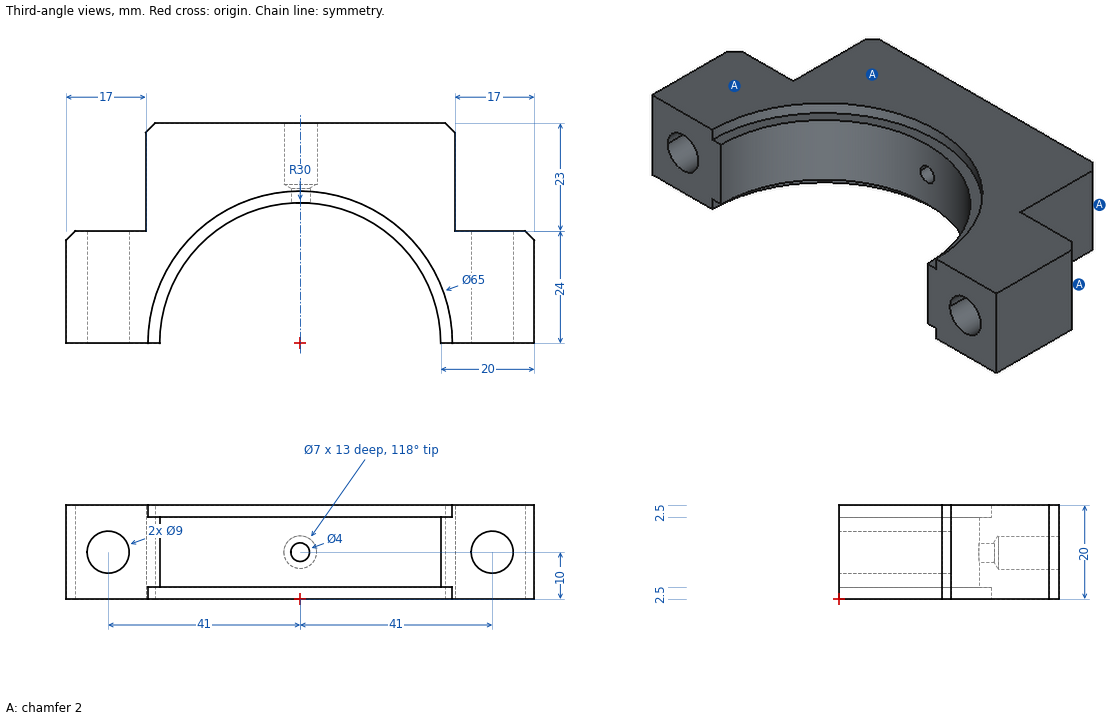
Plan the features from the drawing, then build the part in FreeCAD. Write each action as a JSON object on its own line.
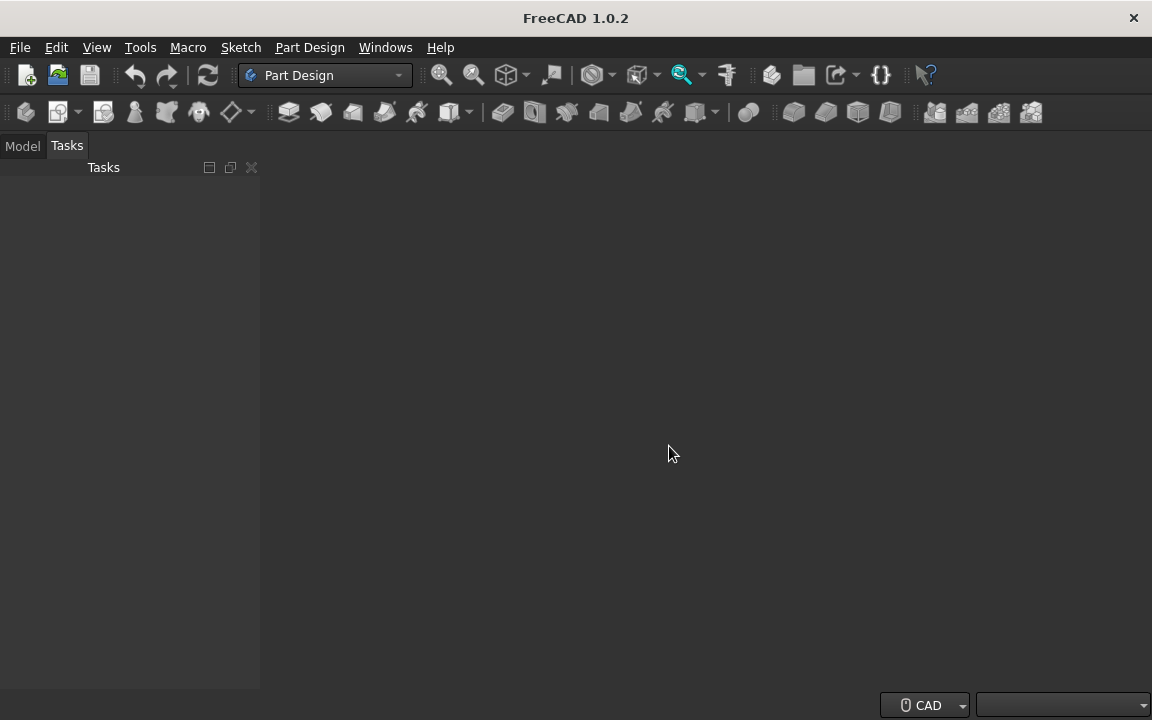
{"action": "left_click", "coordinate": [26, 76]}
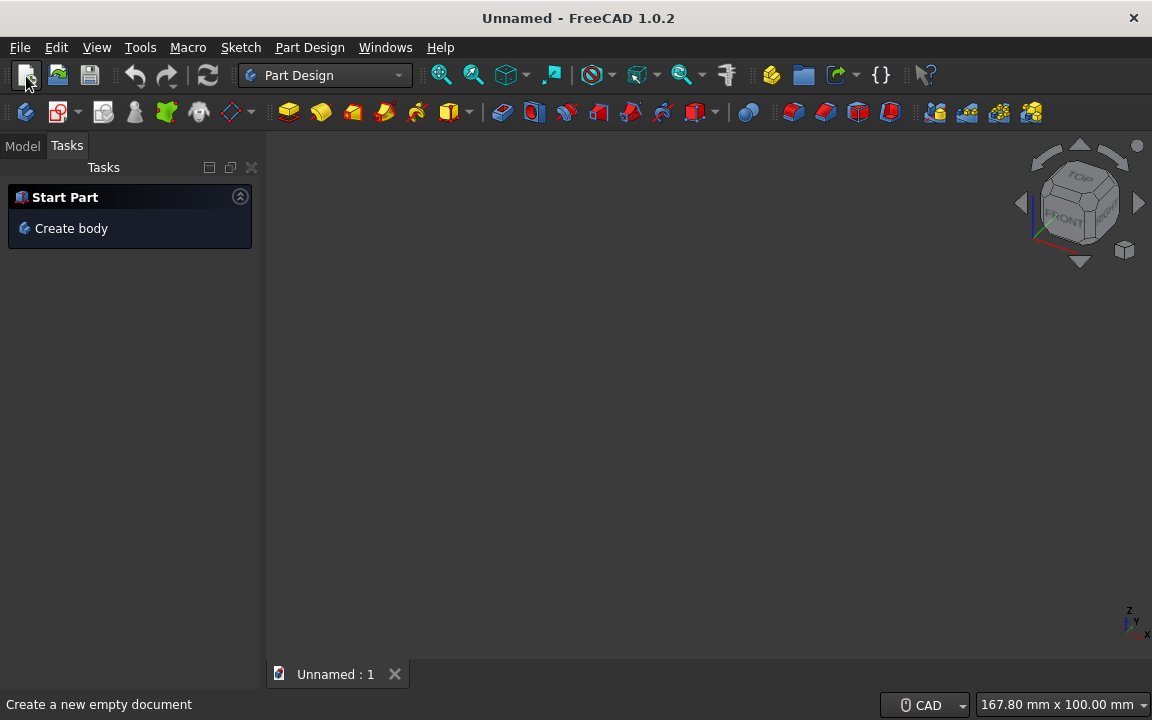
{"action": "left_click", "coordinate": [58, 112]}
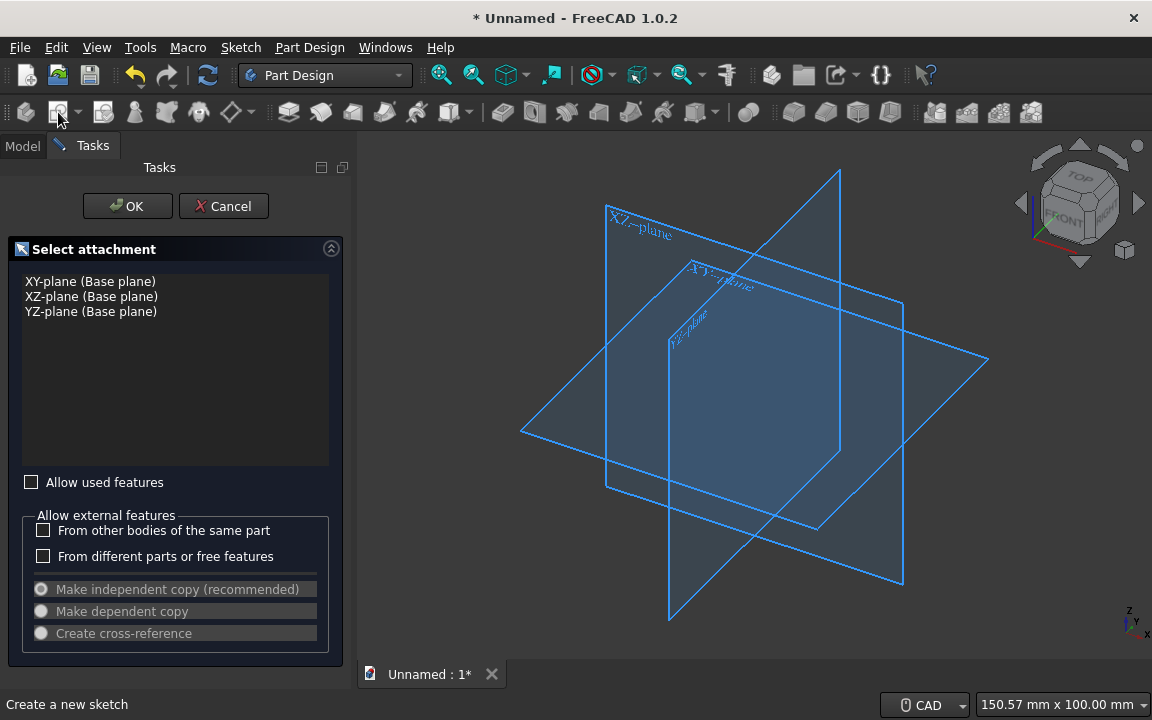
{"action": "left_click", "coordinate": [82, 282]}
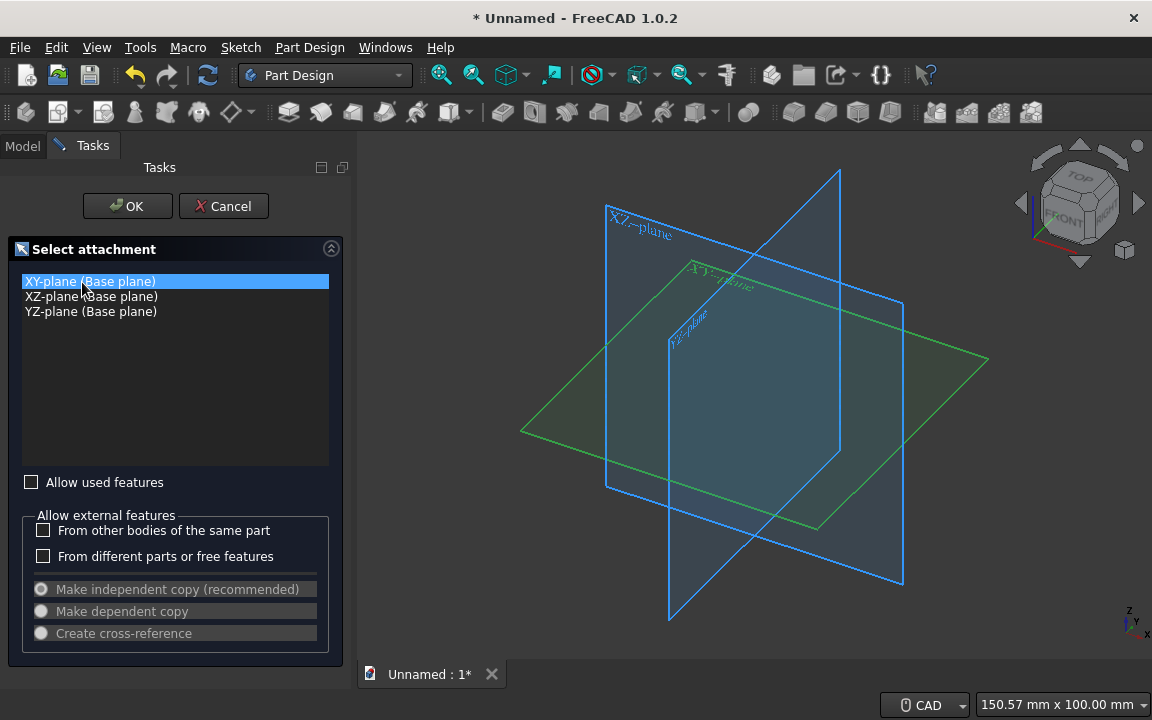
{"action": "left_click", "coordinate": [128, 206]}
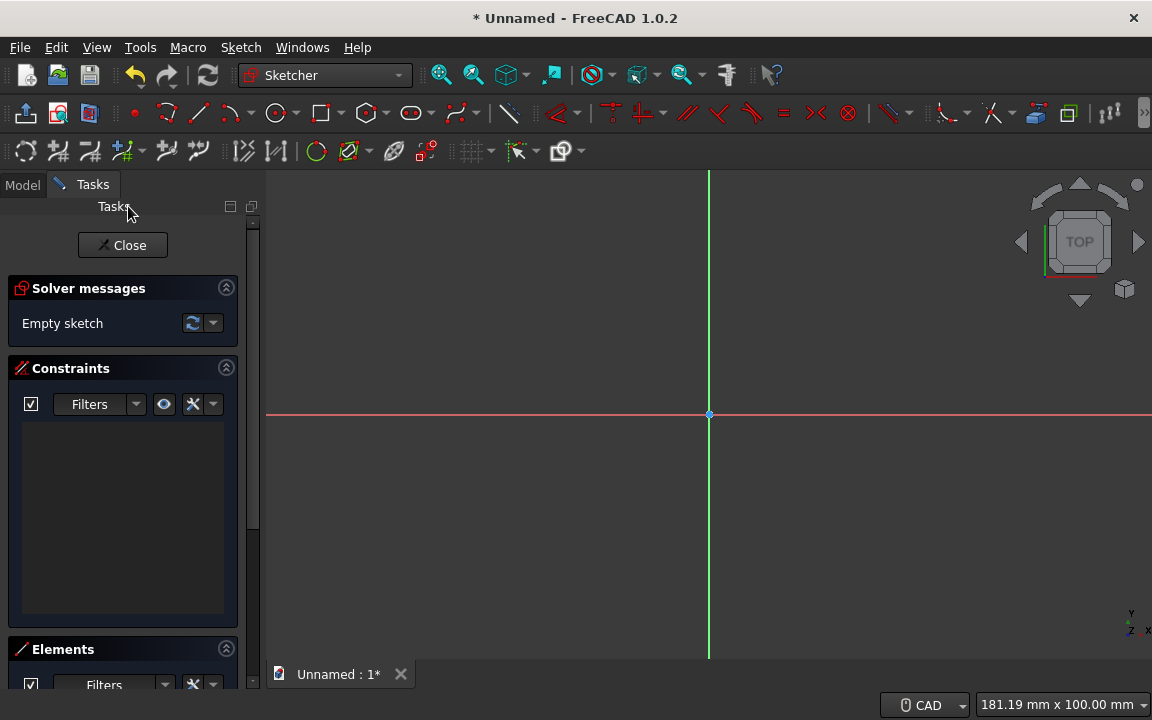
{"action": "scroll", "coordinate": [331, 631], "scroll_direction": "down", "scroll_amount": 1}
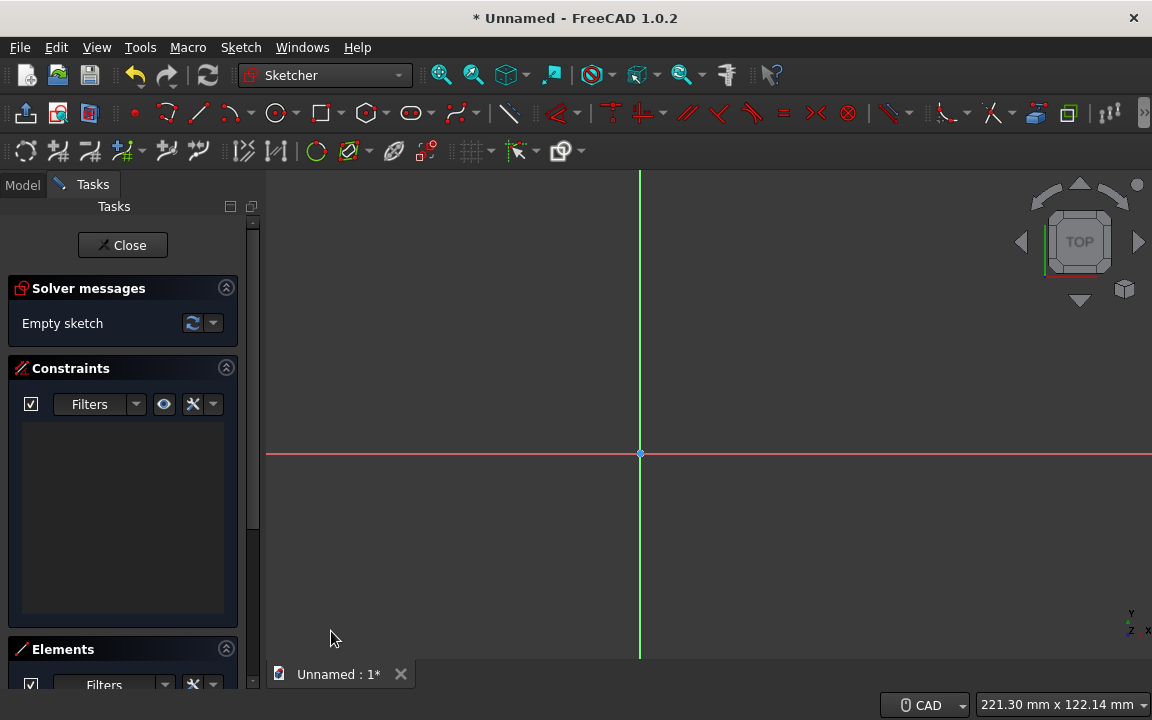
{"action": "left_click", "coordinate": [168, 114]}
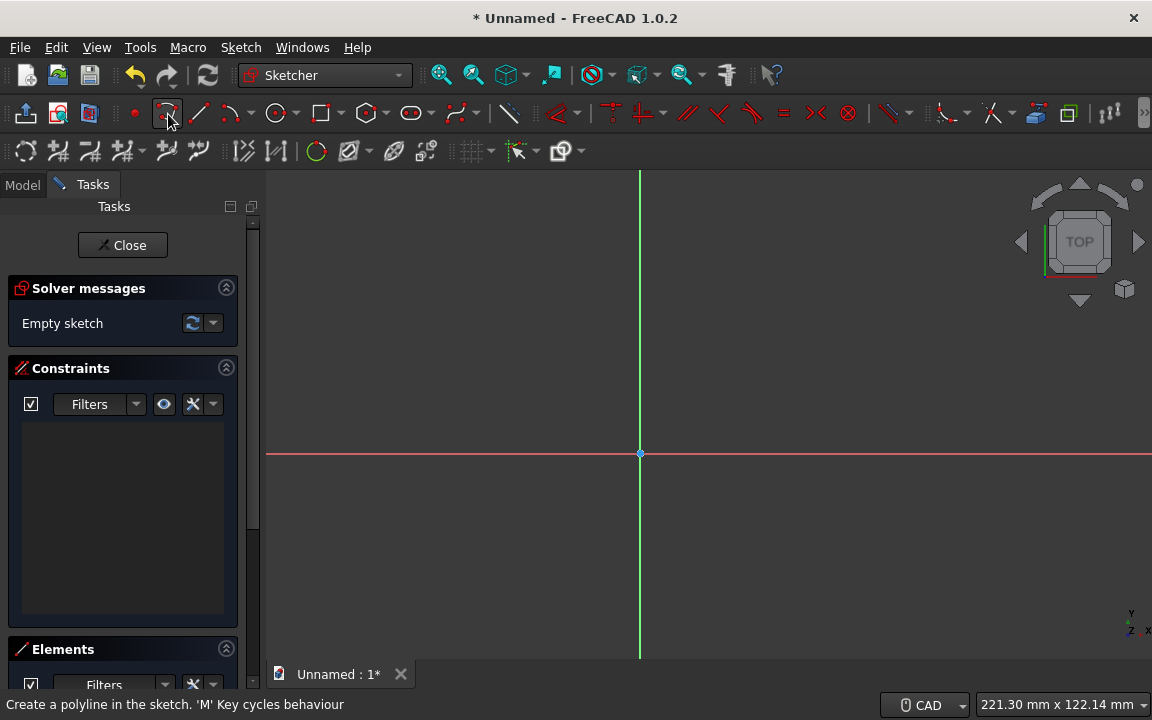
{"action": "left_click", "coordinate": [761, 454]}
{"action": "left_click", "coordinate": [841, 445]}
{"action": "left_click", "coordinate": [841, 358]}
{"action": "left_click", "coordinate": [773, 358]}
{"action": "left_click", "coordinate": [773, 266]}
{"action": "left_click", "coordinate": [508, 266]}
{"action": "left_click", "coordinate": [508, 358]}
{"action": "left_click", "coordinate": [440, 358]}
{"action": "left_click", "coordinate": [440, 454]}
{"action": "left_click", "coordinate": [520, 445]}
{"action": "right_click", "coordinate": [520, 445]}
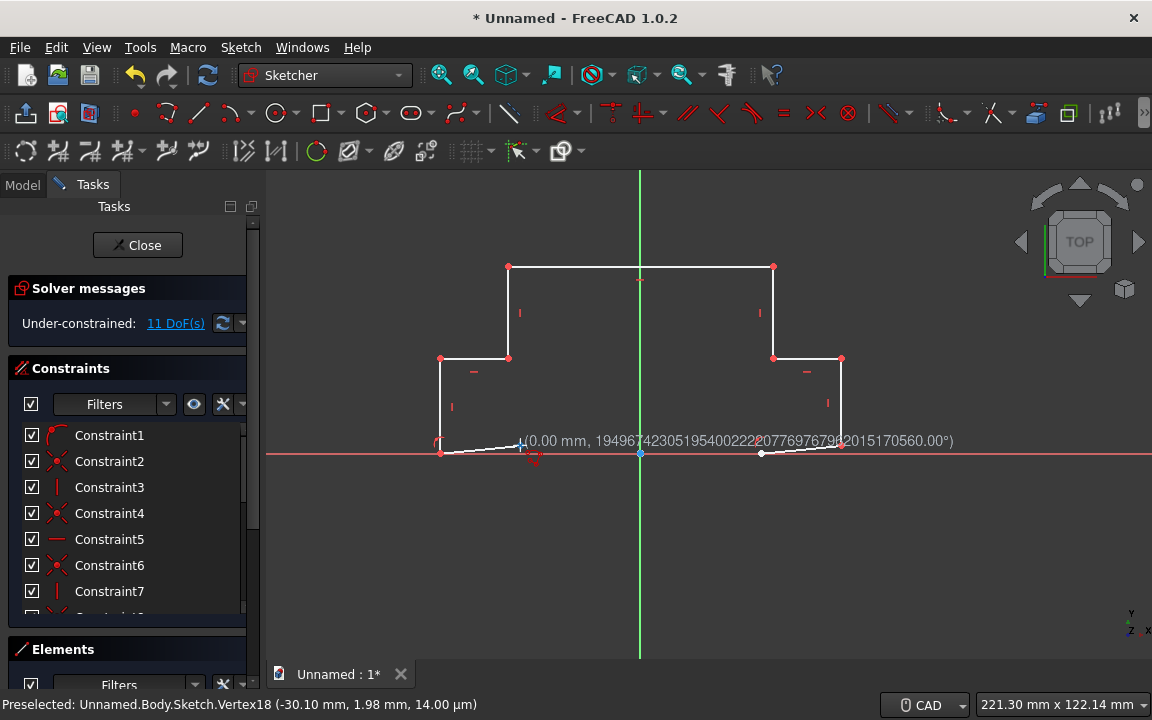
{"action": "key", "text": "g 3 a"}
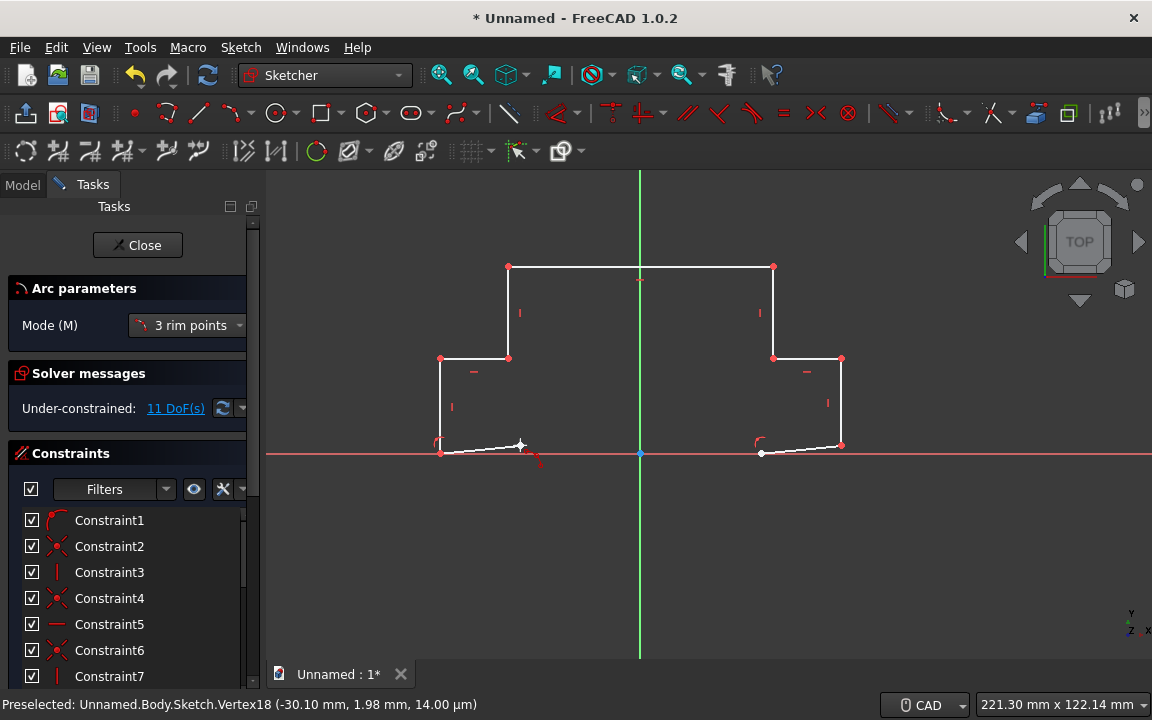
{"action": "left_click", "coordinate": [520, 446]}
{"action": "left_click", "coordinate": [761, 454]}
{"action": "left_click", "coordinate": [678, 340]}
{"action": "key", "text": "Escape"}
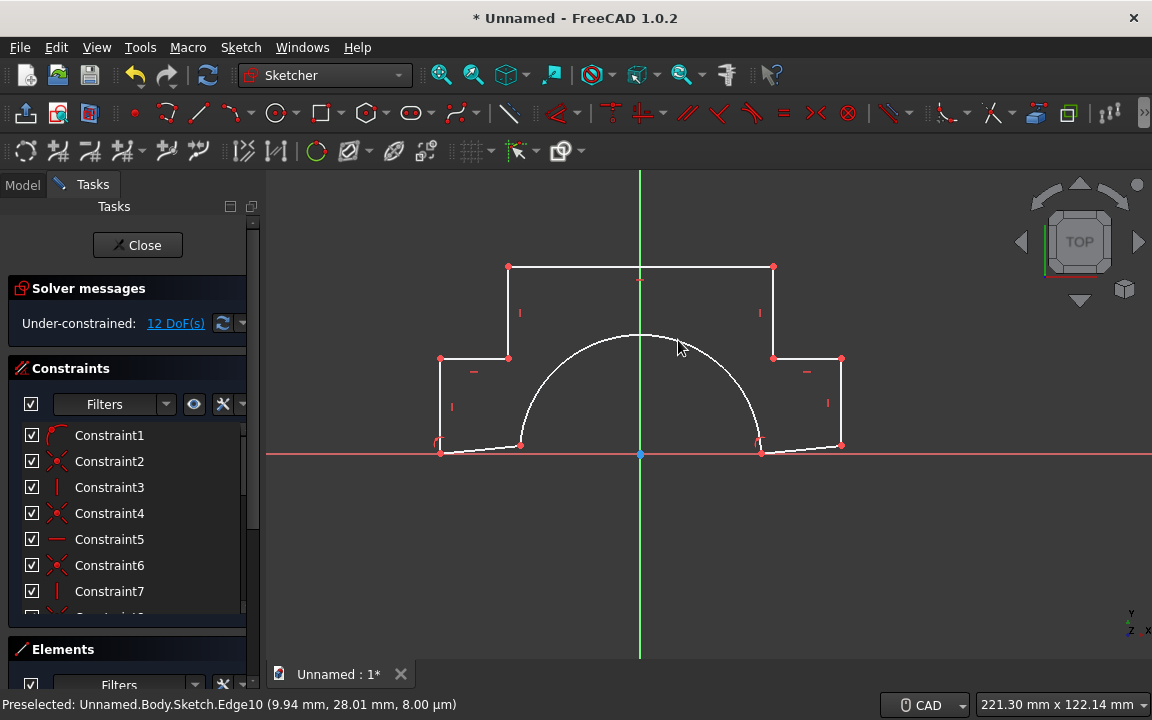
{"action": "left_click", "coordinate": [785, 452]}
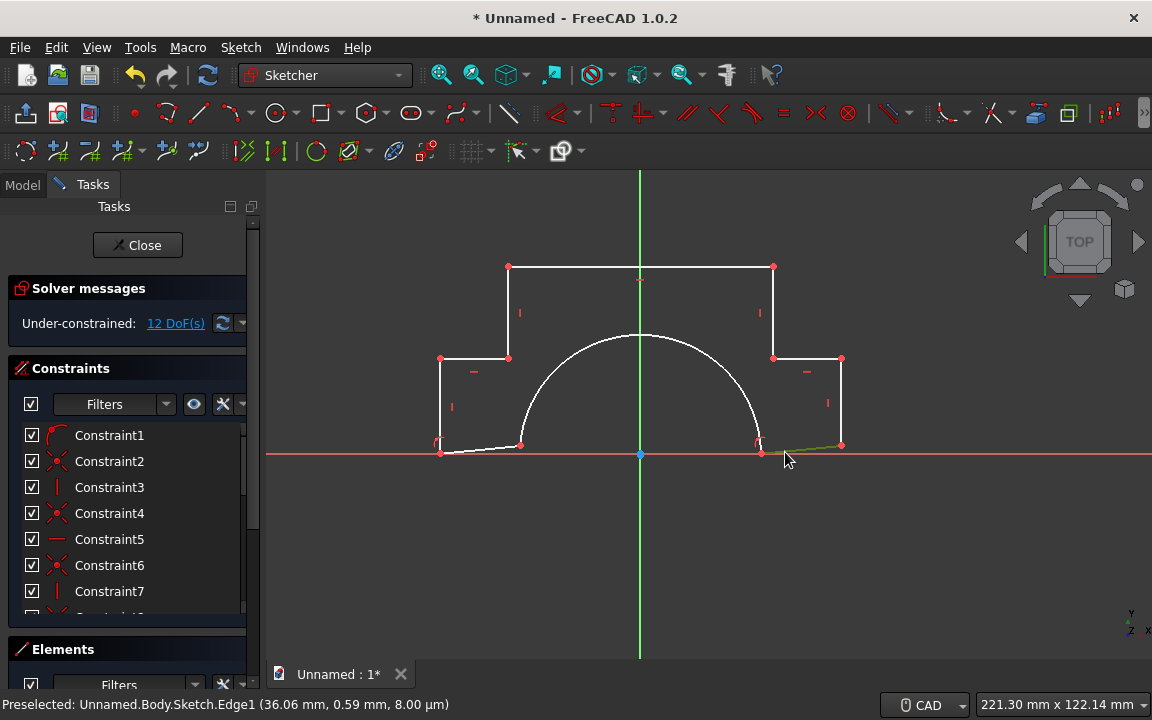
{"action": "left_click", "coordinate": [666, 114]}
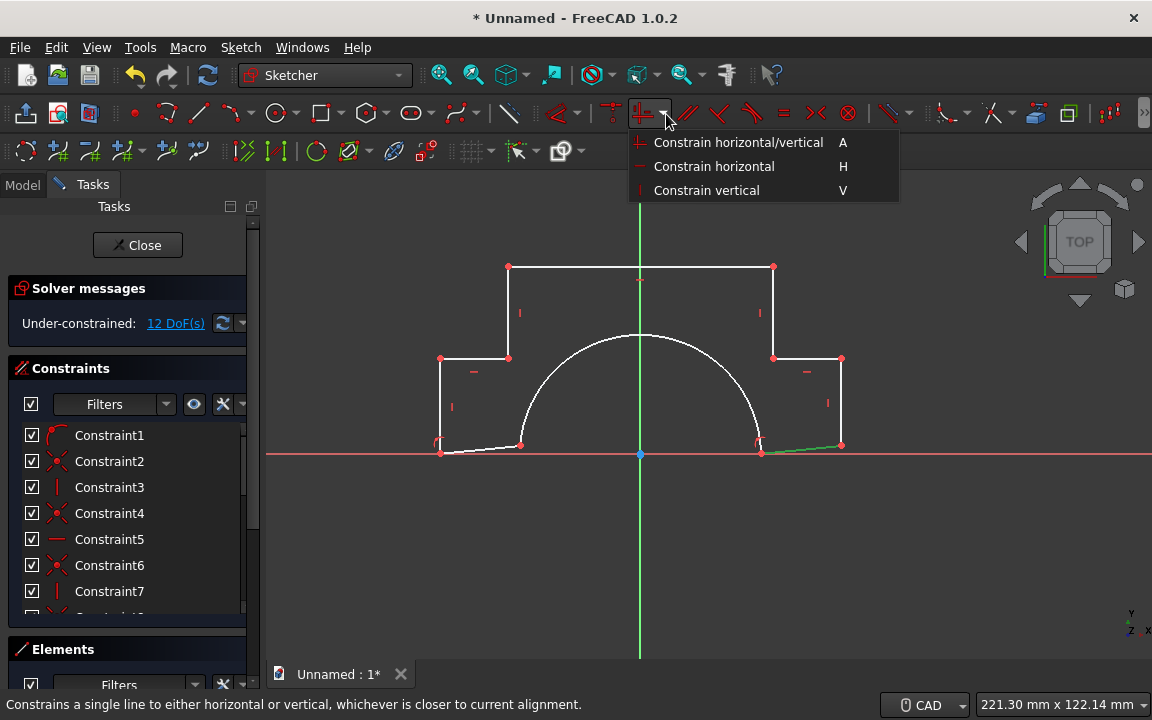
{"action": "left_click", "coordinate": [764, 166]}